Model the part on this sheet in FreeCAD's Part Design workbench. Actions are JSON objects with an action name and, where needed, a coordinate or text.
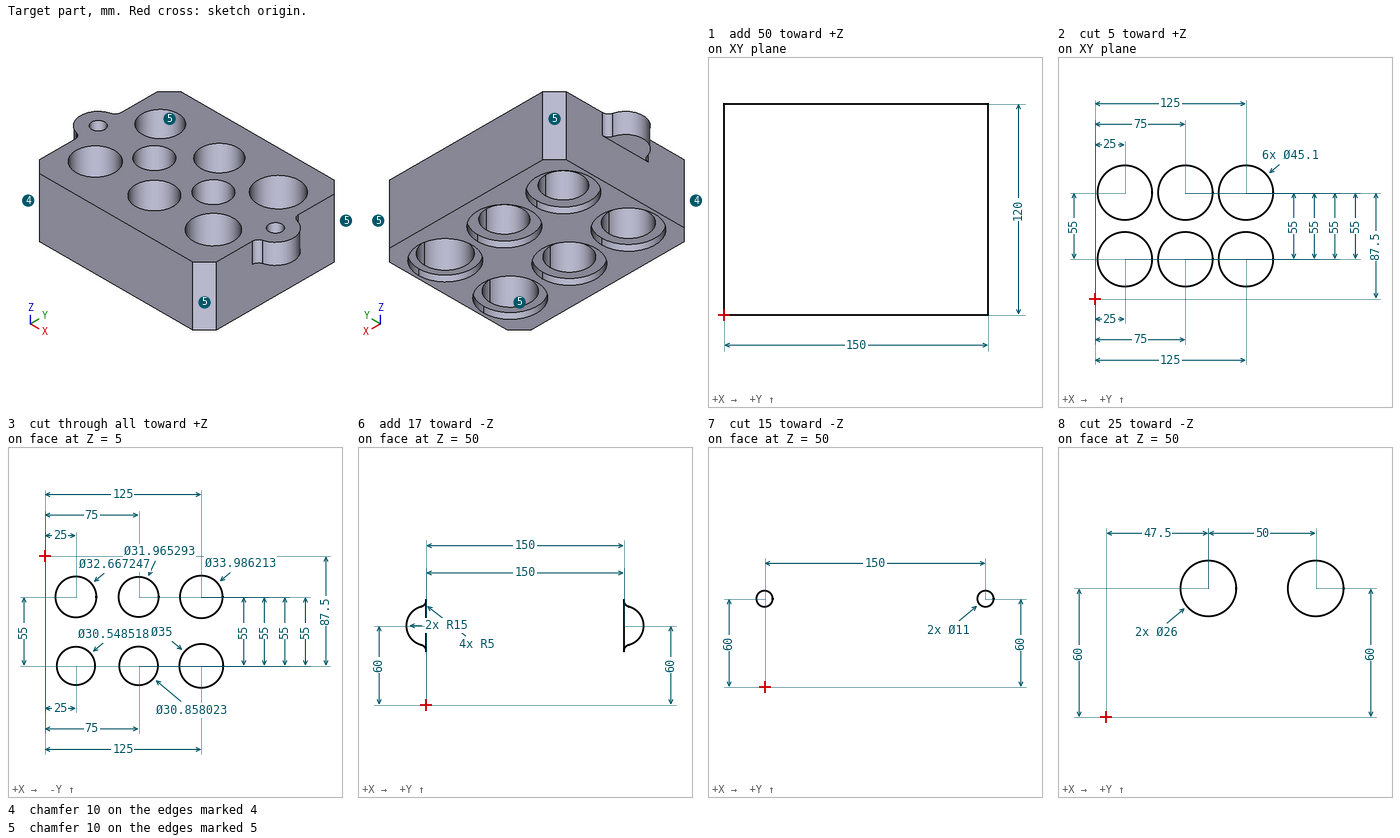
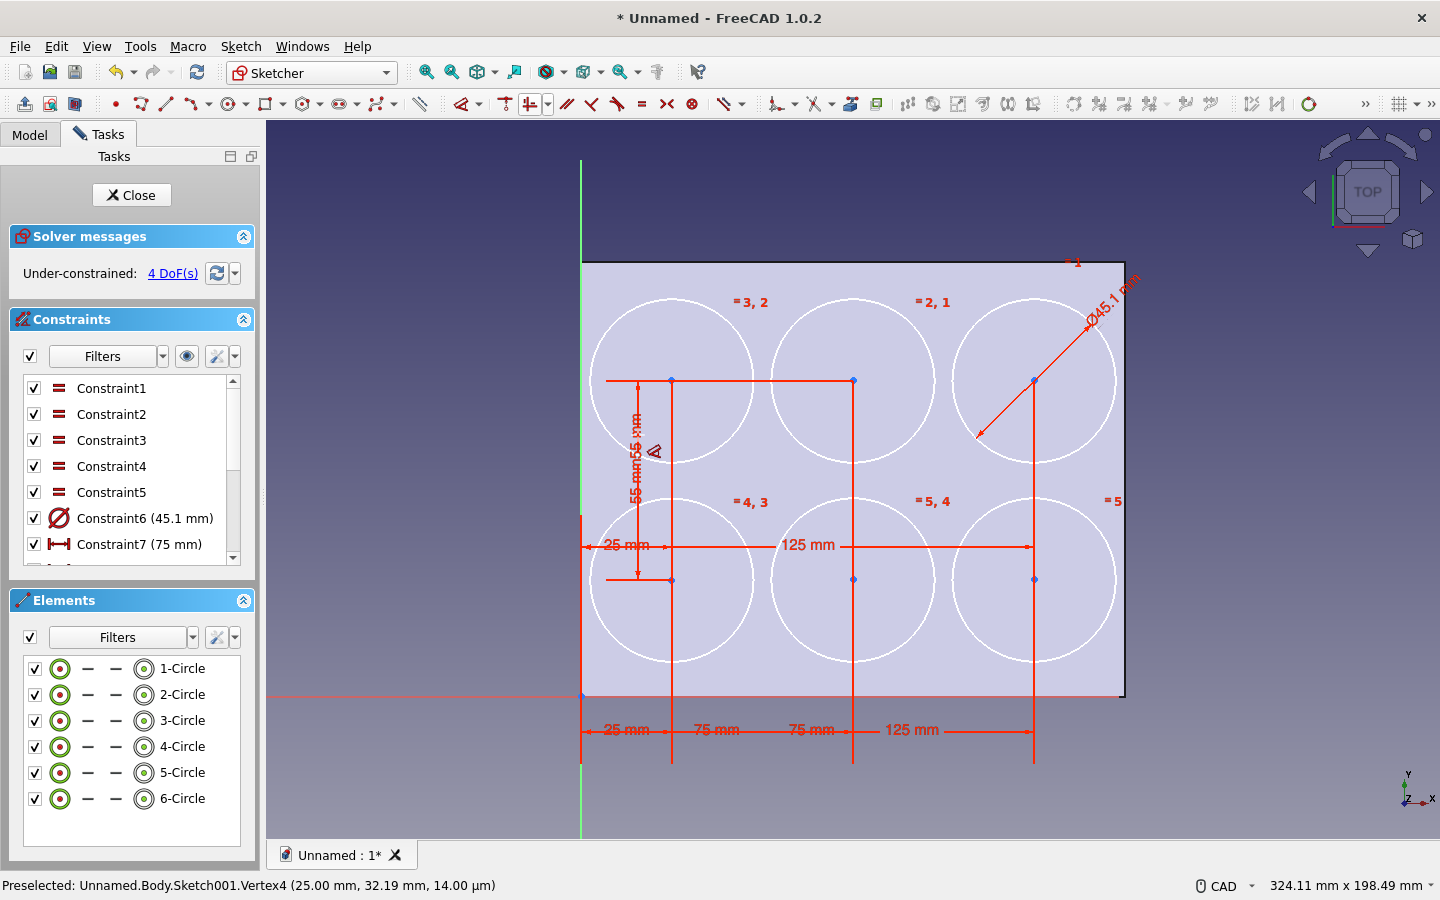
{"action": "left_click", "coordinate": [1034, 381]}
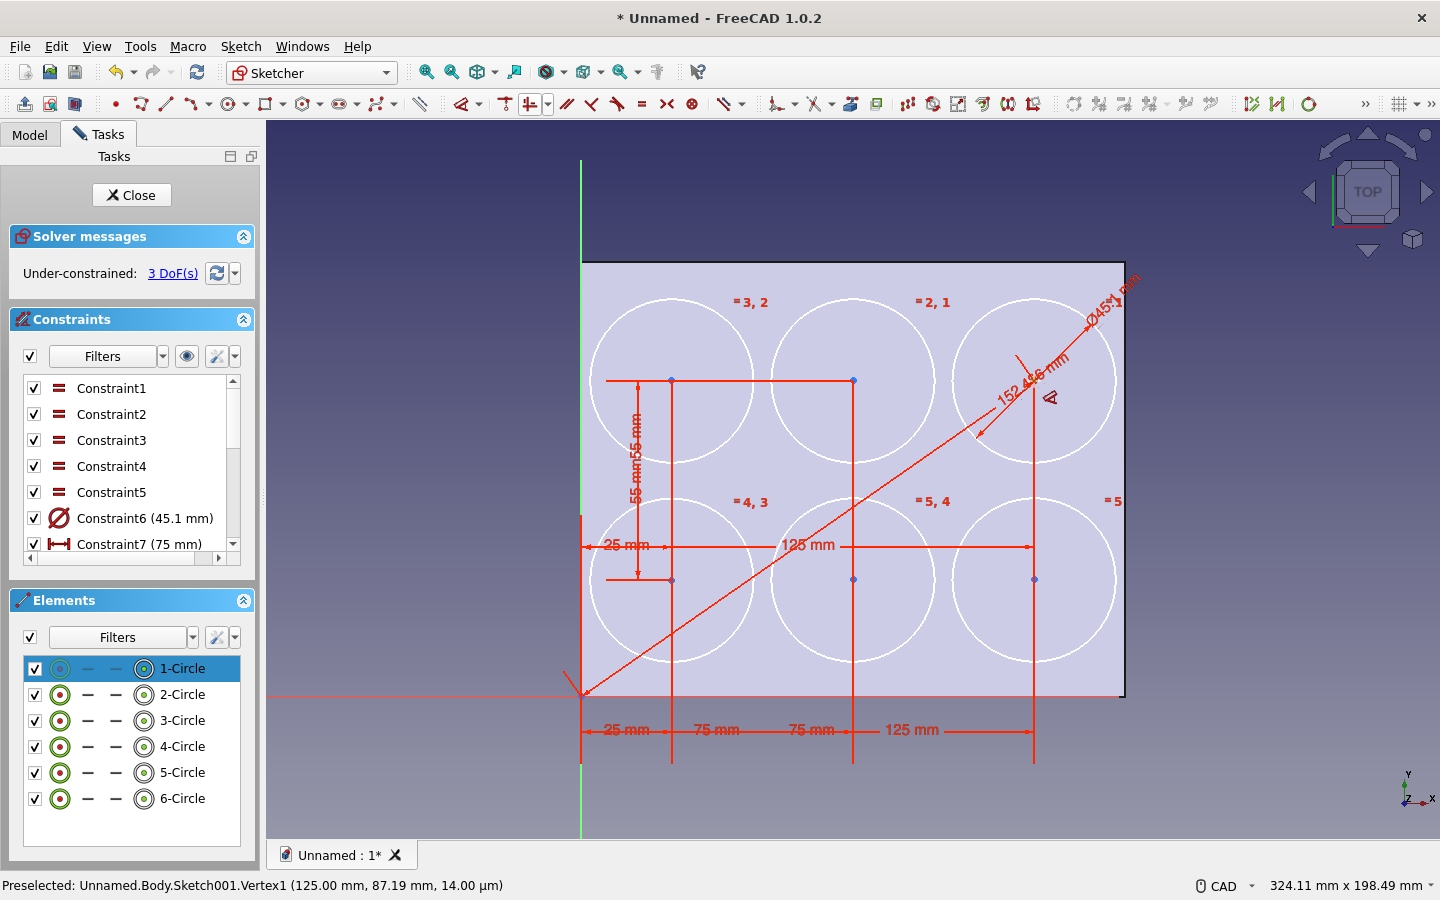
{"action": "left_click", "coordinate": [672, 580]}
{"action": "left_click", "coordinate": [1068, 481]}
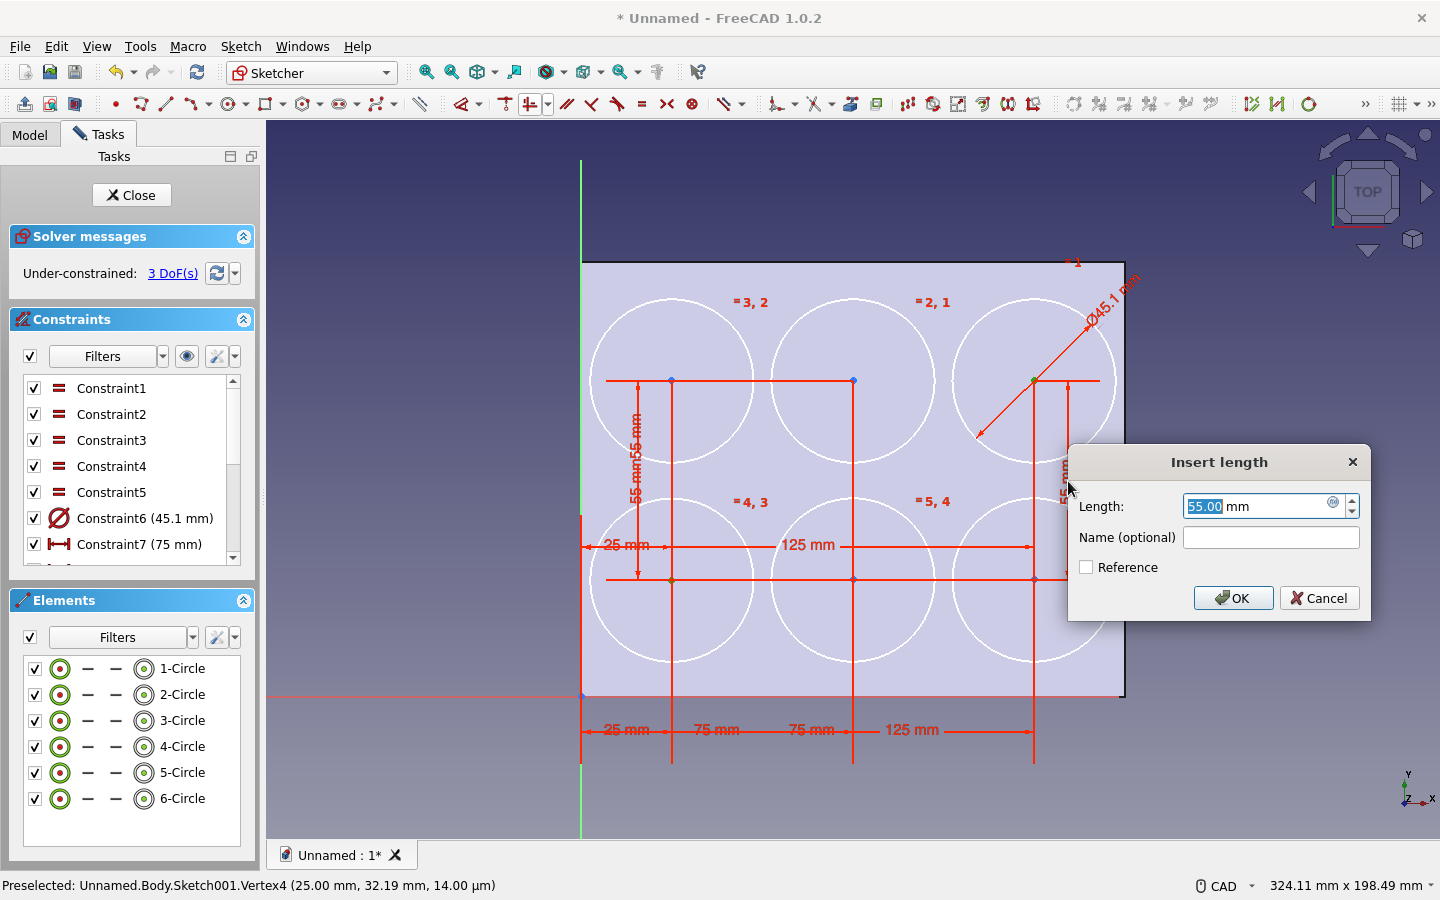
{"action": "type", "text": "55"}
{"action": "key", "text": "Return"}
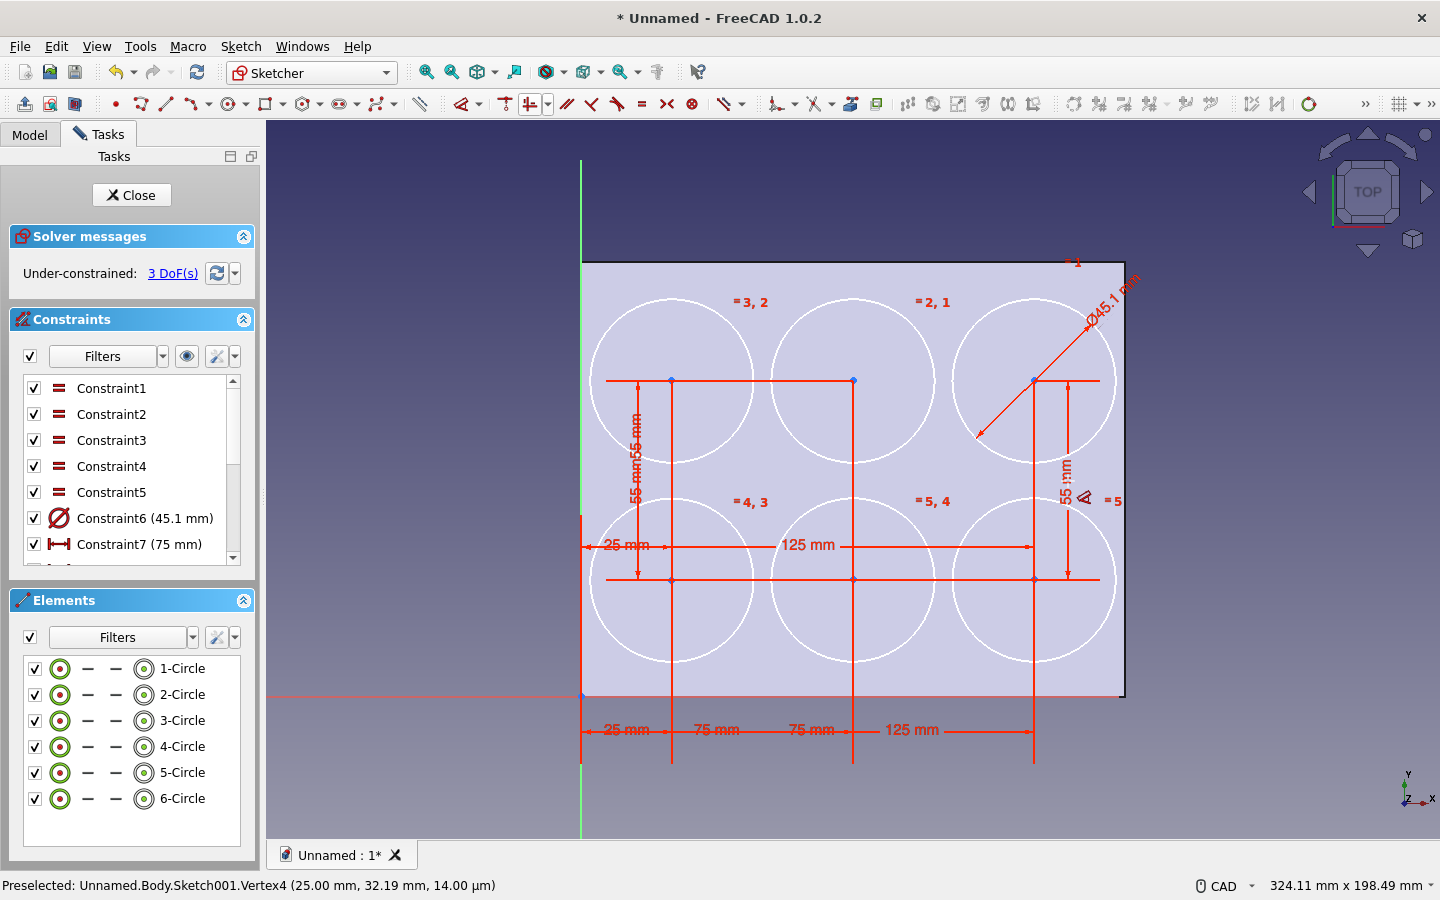
{"action": "left_click", "coordinate": [853, 381]}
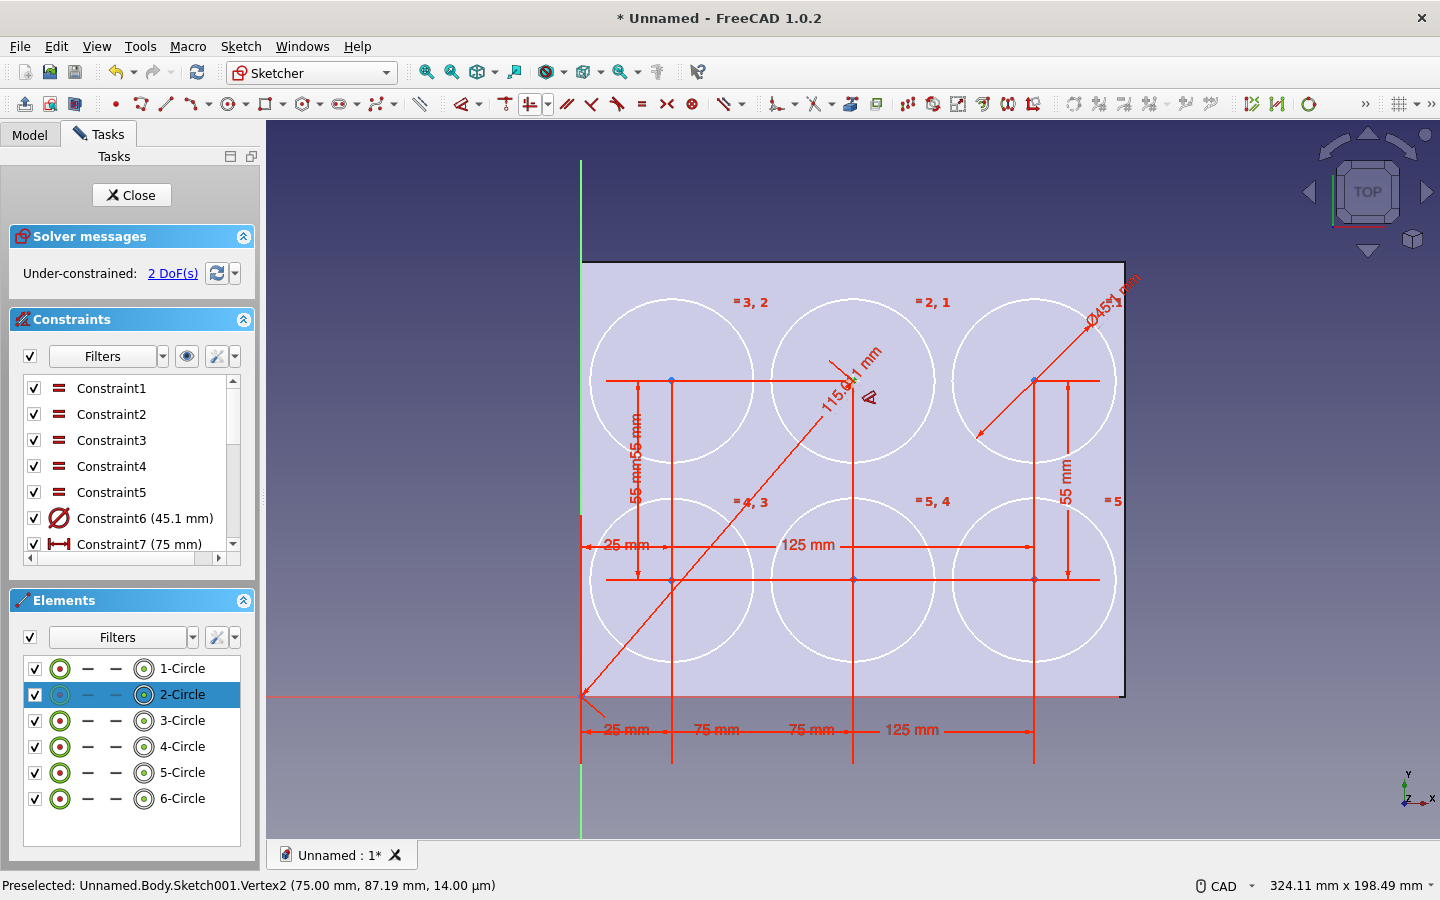
{"action": "left_click", "coordinate": [853, 580]}
{"action": "left_click", "coordinate": [887, 480]}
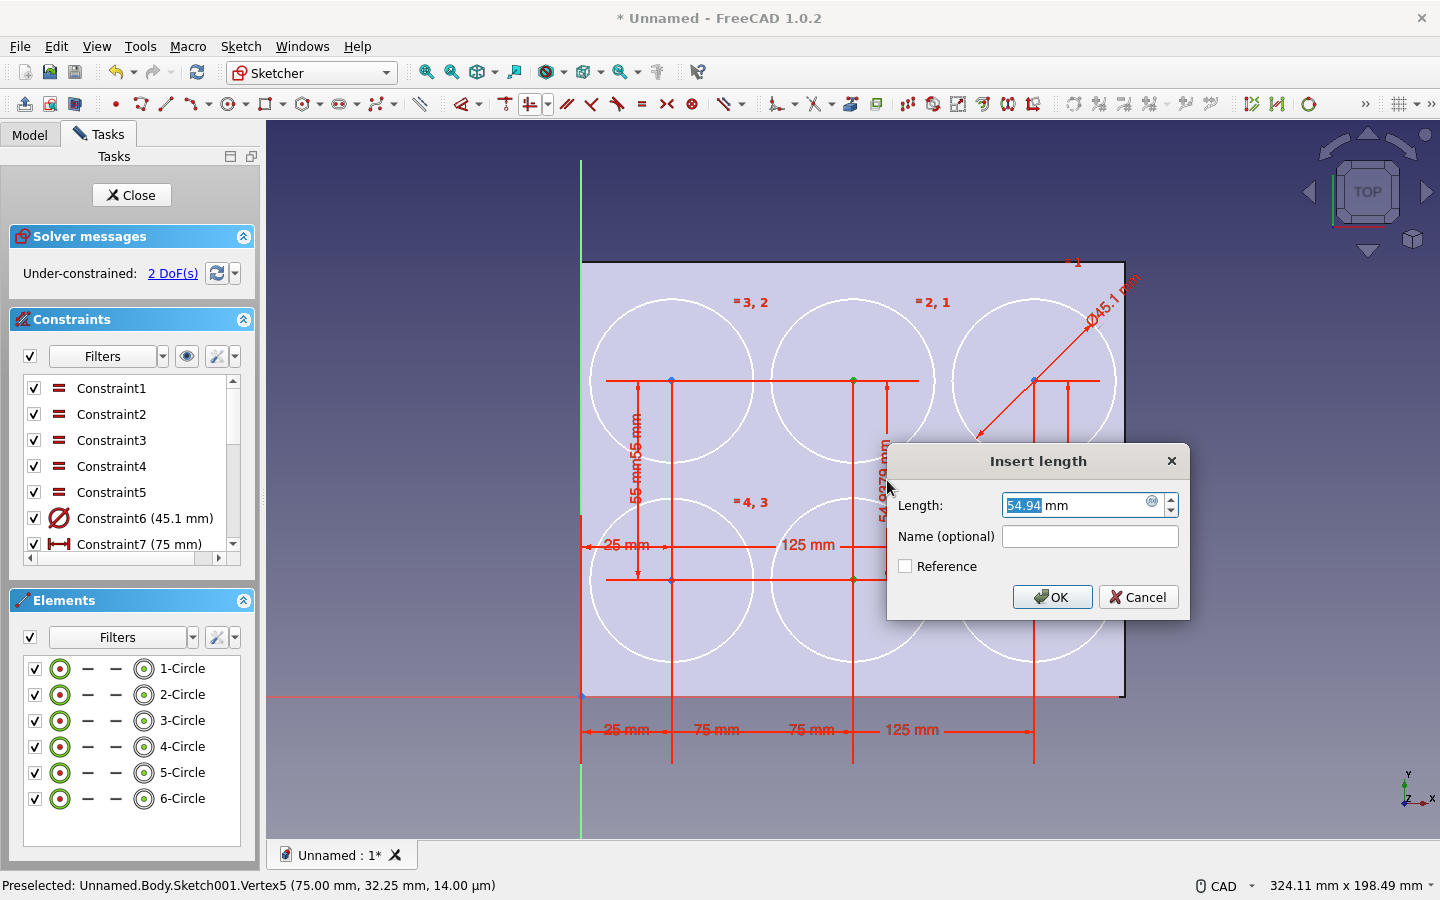
{"action": "type", "text": "55"}
{"action": "key", "text": "Return"}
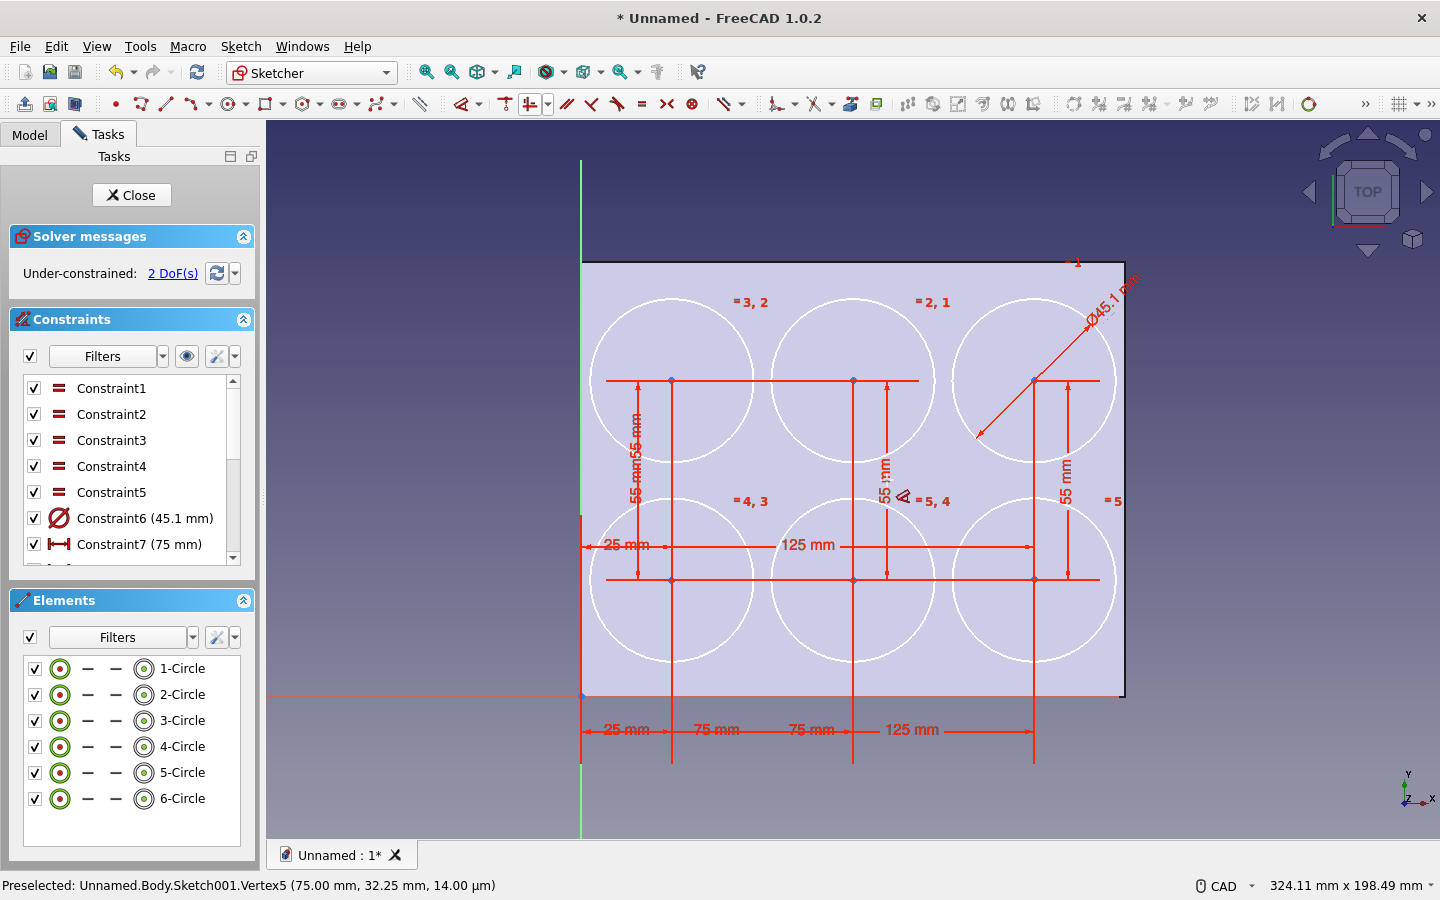
{"action": "left_click", "coordinate": [1034, 381]}